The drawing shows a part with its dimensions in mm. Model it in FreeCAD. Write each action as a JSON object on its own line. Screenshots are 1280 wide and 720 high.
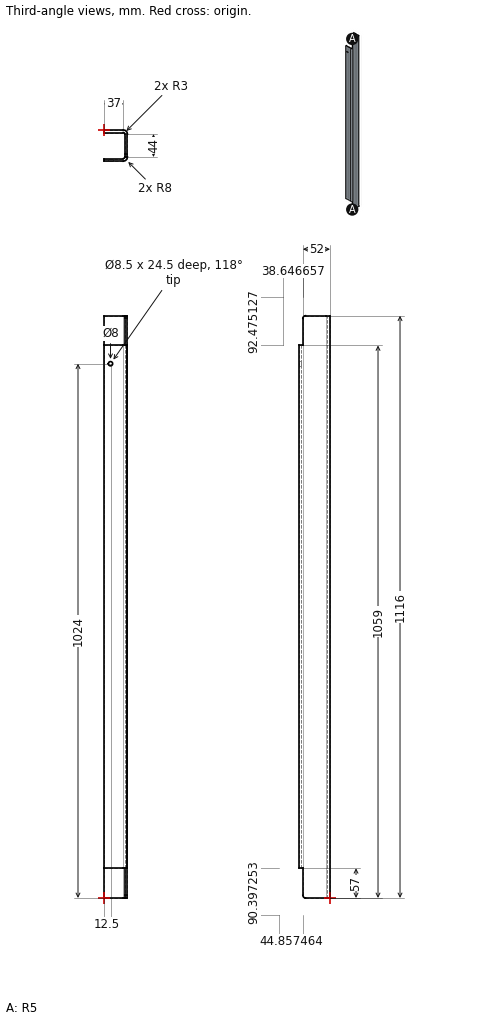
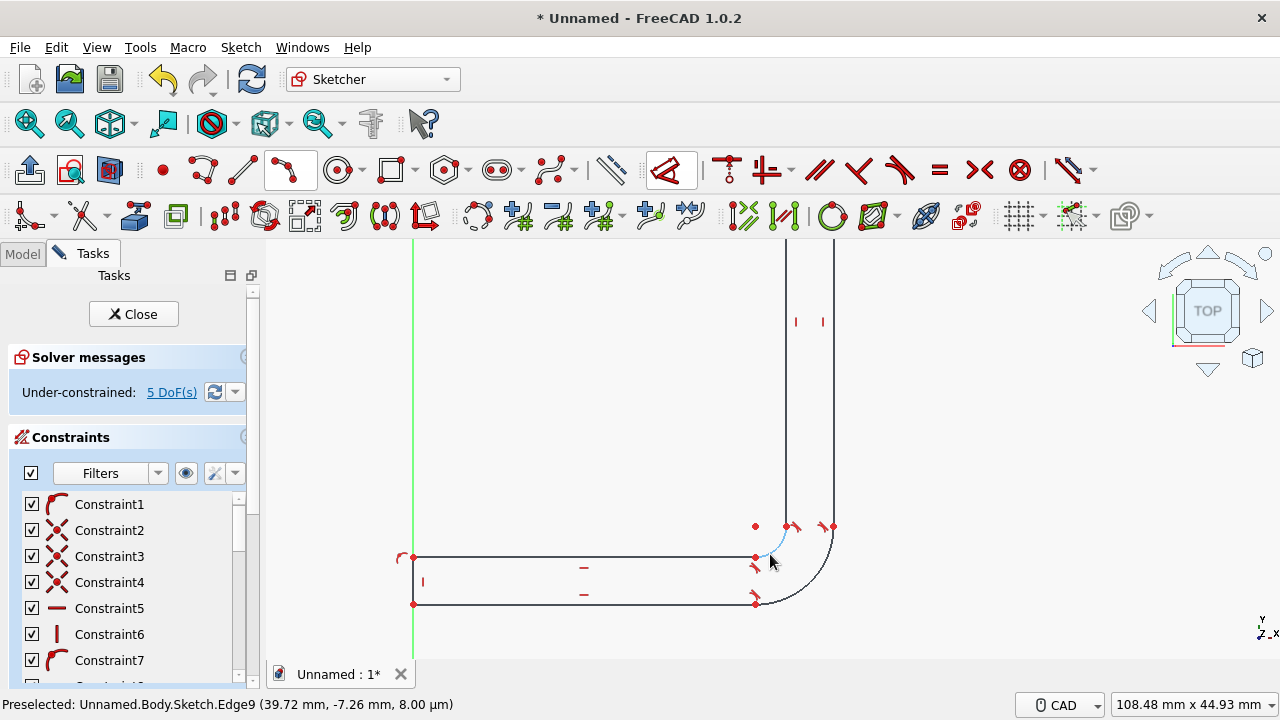
{"action": "left_click", "coordinate": [769, 554]}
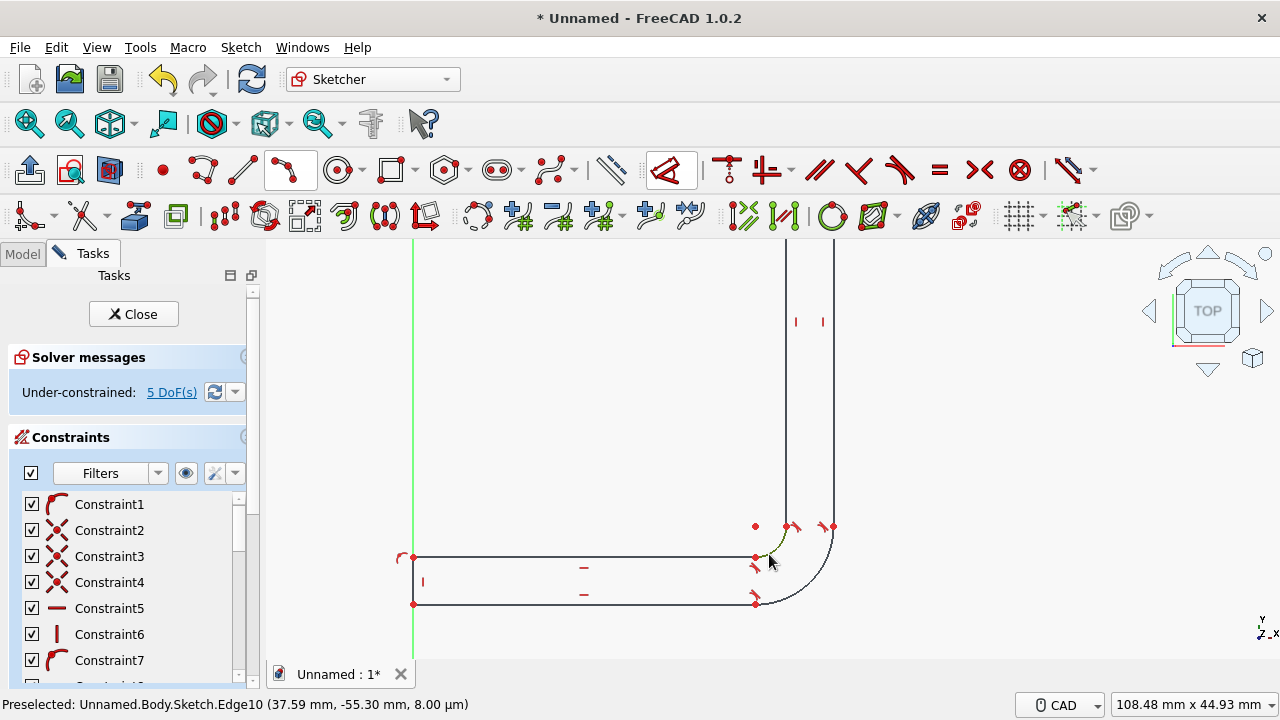
{"action": "left_click", "coordinate": [940, 170]}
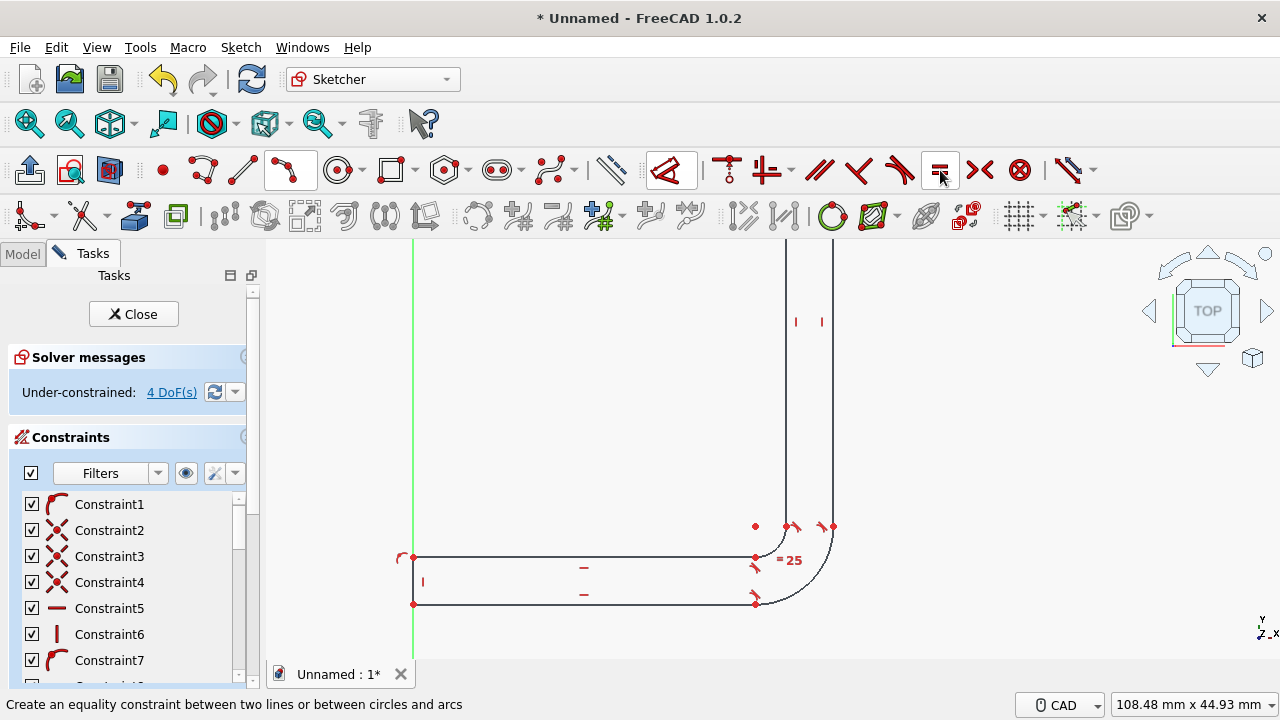
{"action": "key", "text": "d"}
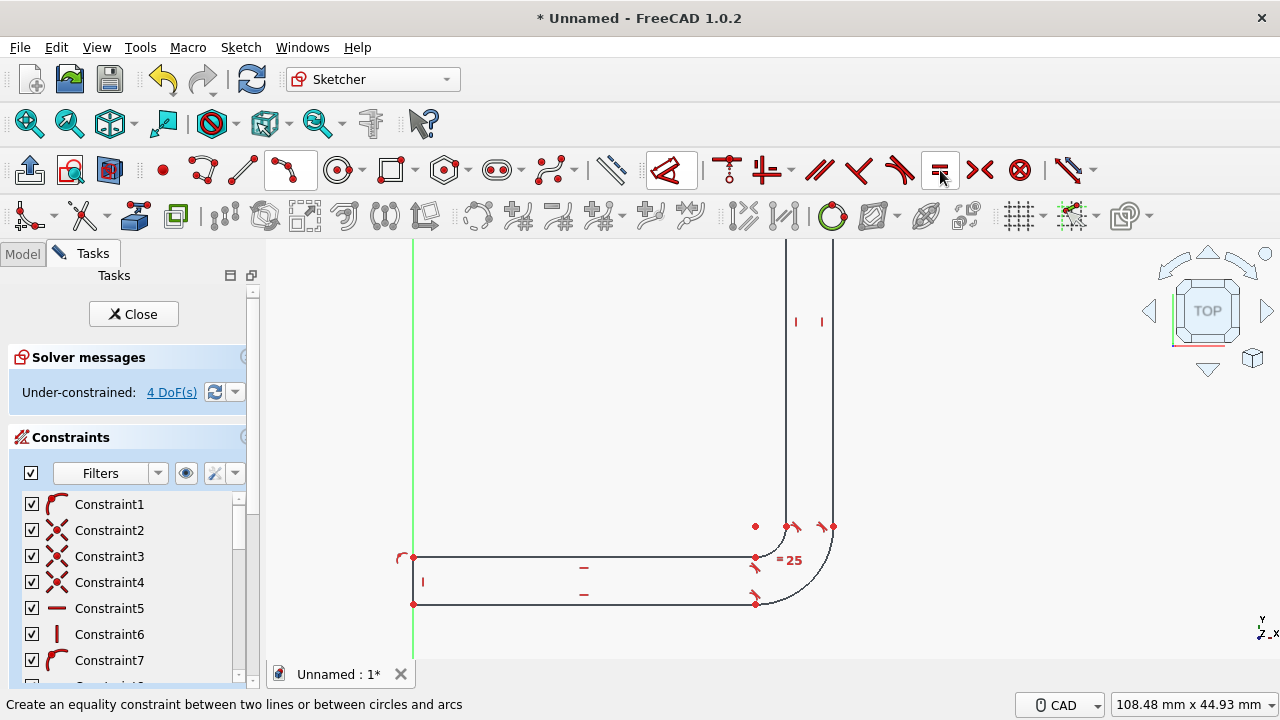
{"action": "scroll", "coordinate": [770, 555], "scroll_direction": "down", "scroll_amount": 4}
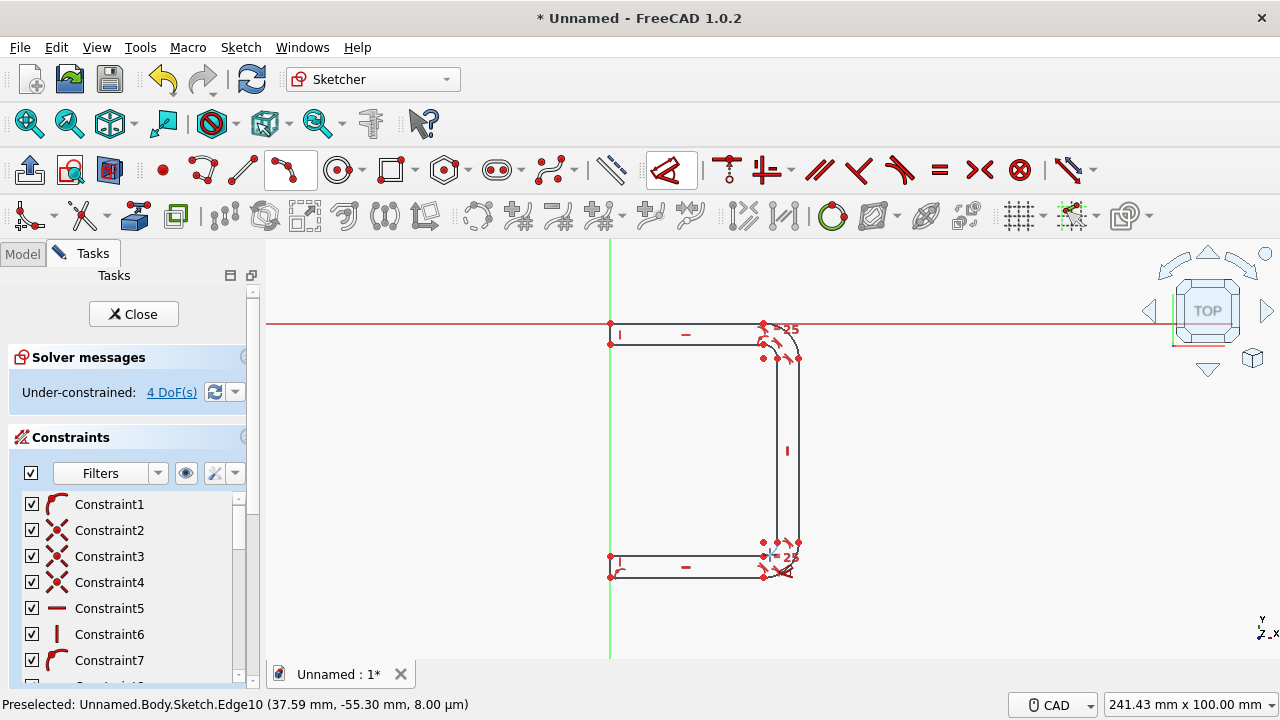
{"action": "scroll", "coordinate": [776, 352], "scroll_direction": "up", "scroll_amount": 6}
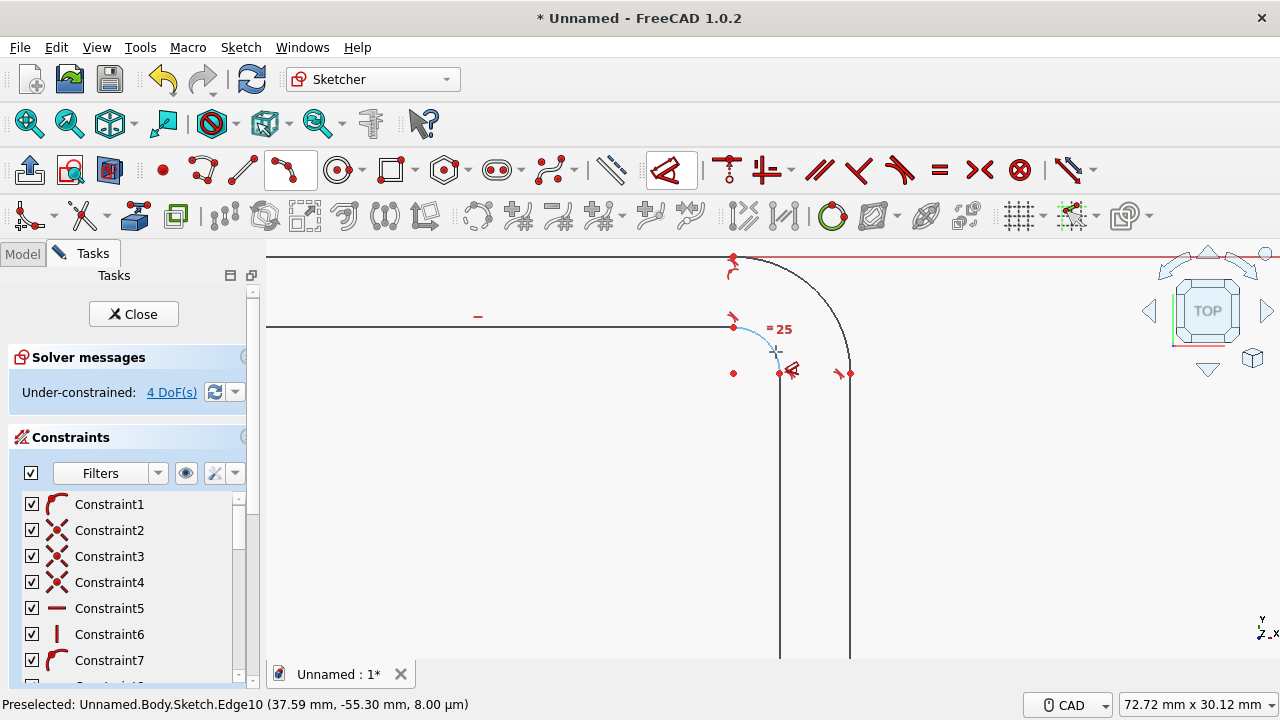
{"action": "left_click", "coordinate": [775, 353]}
{"action": "left_click", "coordinate": [804, 339]}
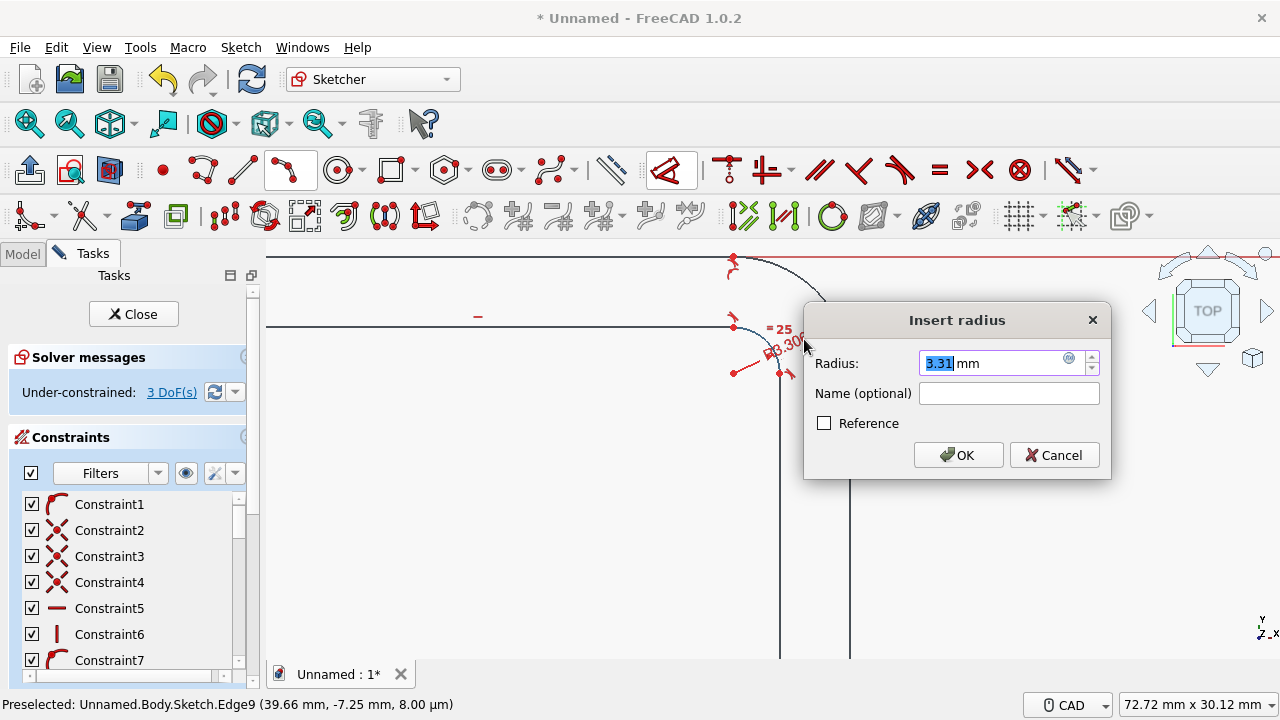
{"action": "type", "text": "3"}
{"action": "key", "text": "Return"}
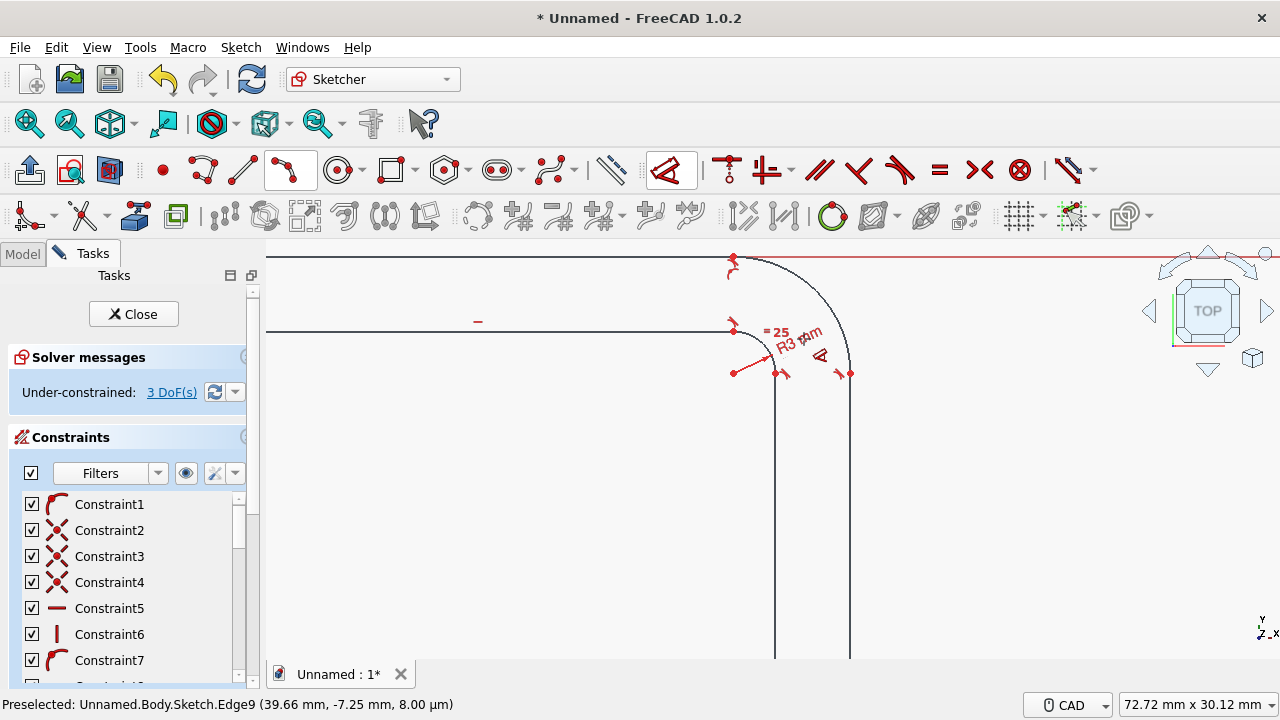
{"action": "scroll", "coordinate": [776, 352], "scroll_direction": "down", "scroll_amount": 6}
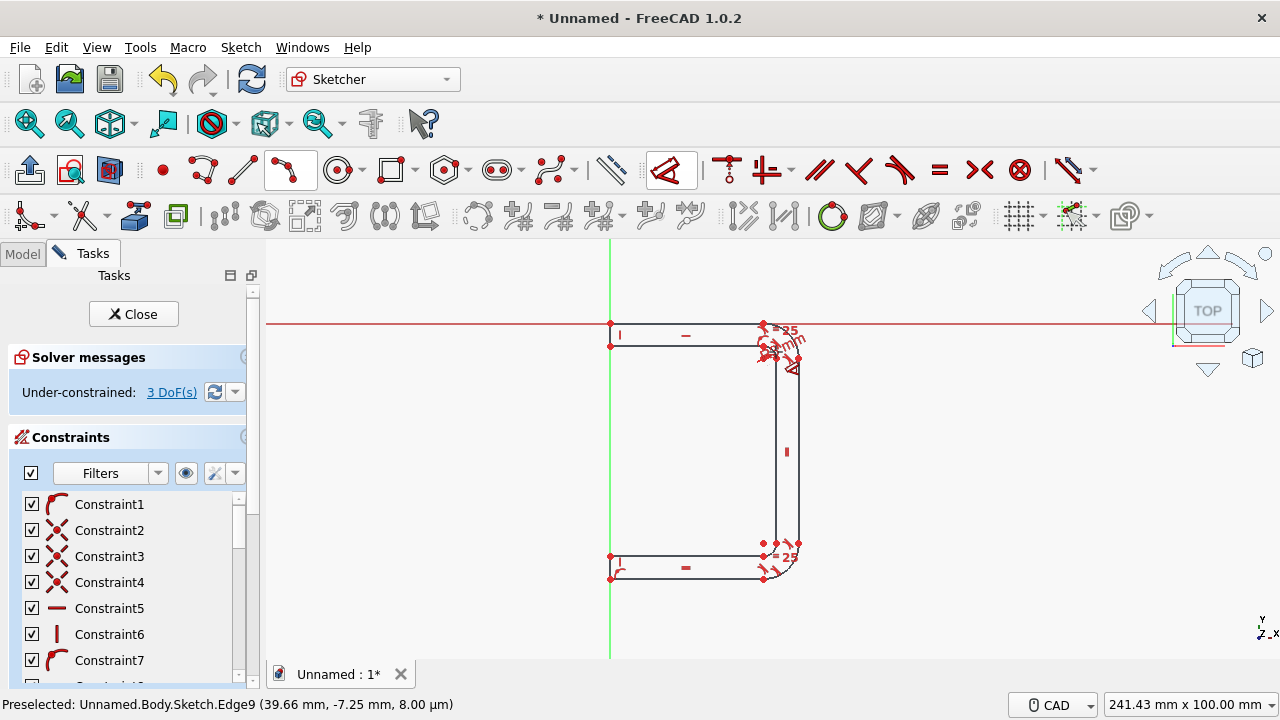
{"action": "left_click", "coordinate": [780, 575]}
{"action": "left_click", "coordinate": [795, 603]}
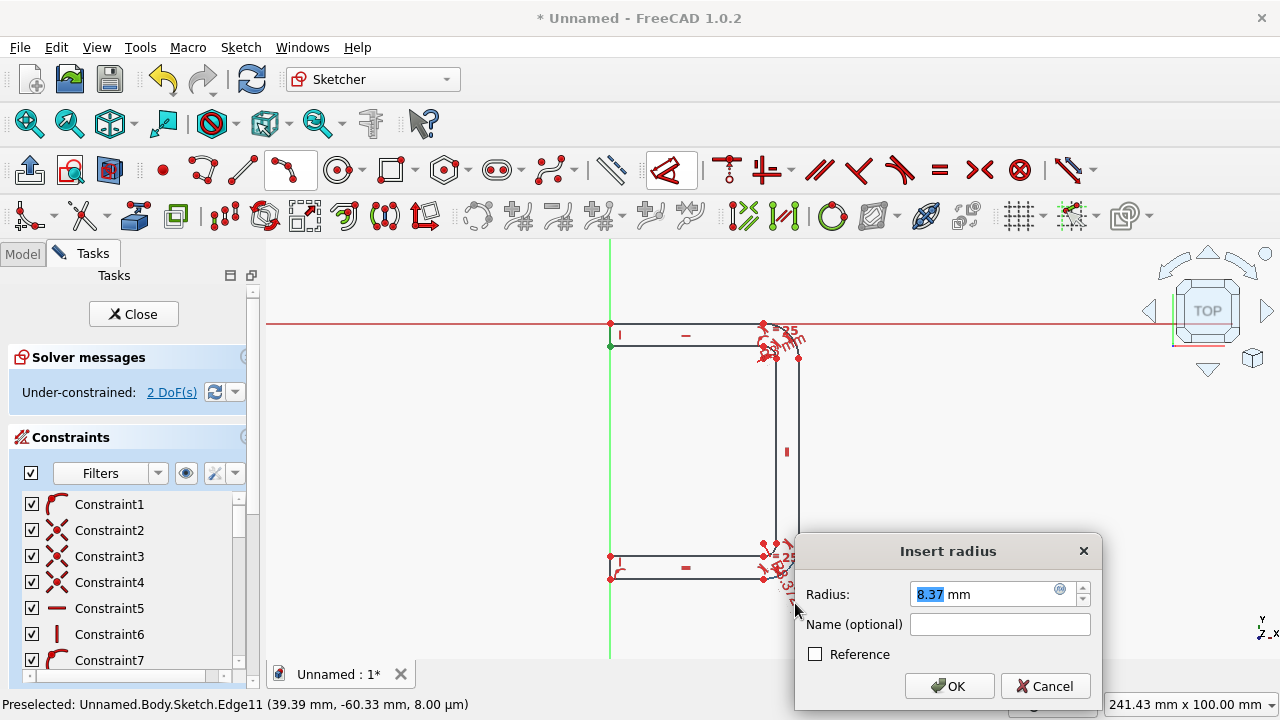
{"action": "type", "text": "8"}
{"action": "key", "text": "Return"}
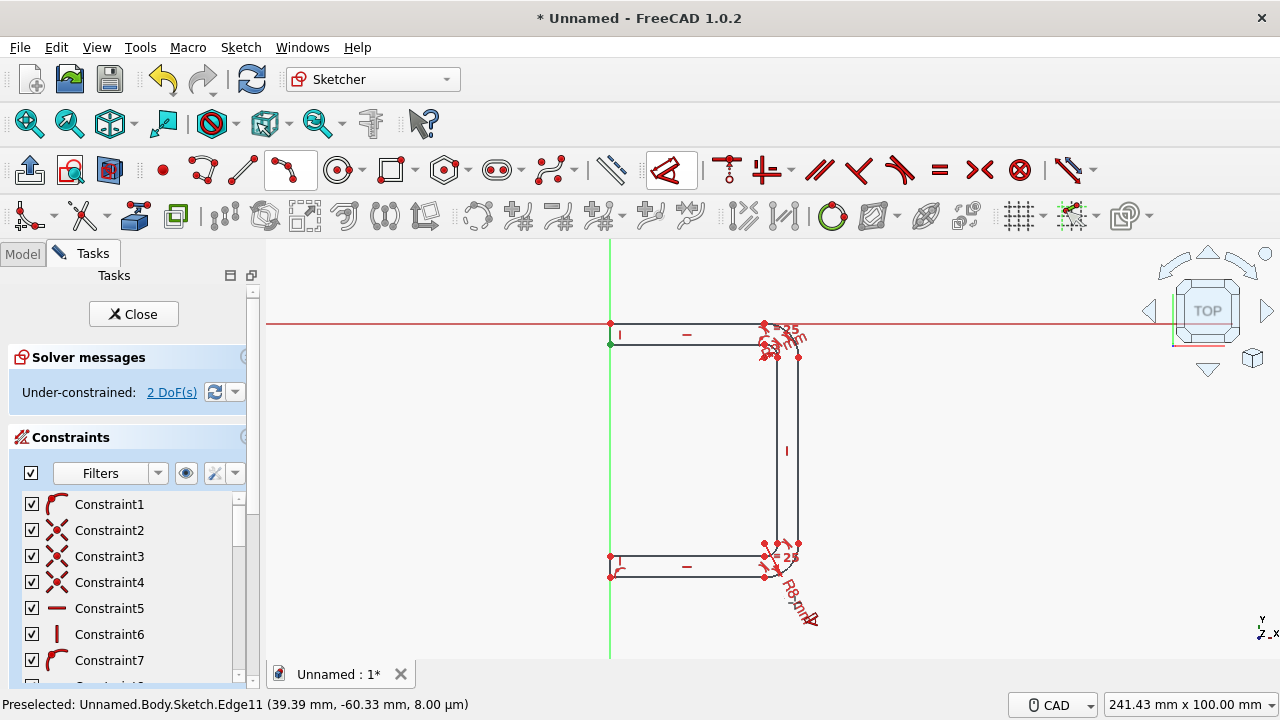
{"action": "left_click", "coordinate": [718, 324]}
{"action": "left_click", "coordinate": [687, 290]}